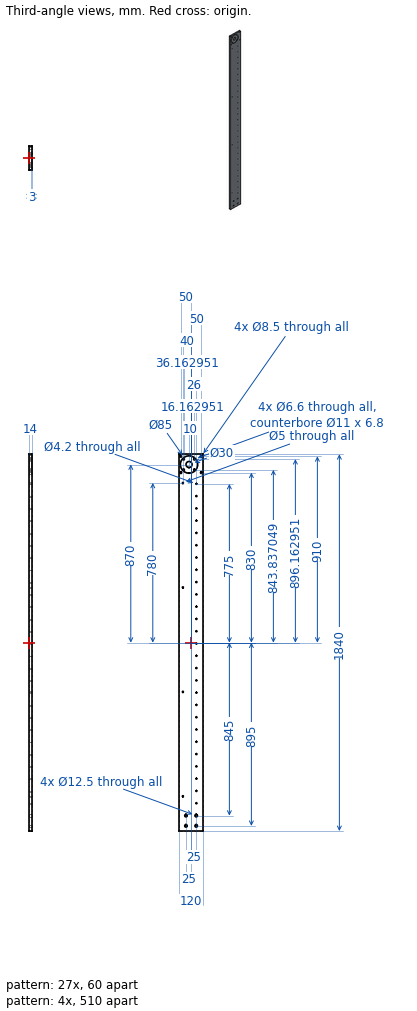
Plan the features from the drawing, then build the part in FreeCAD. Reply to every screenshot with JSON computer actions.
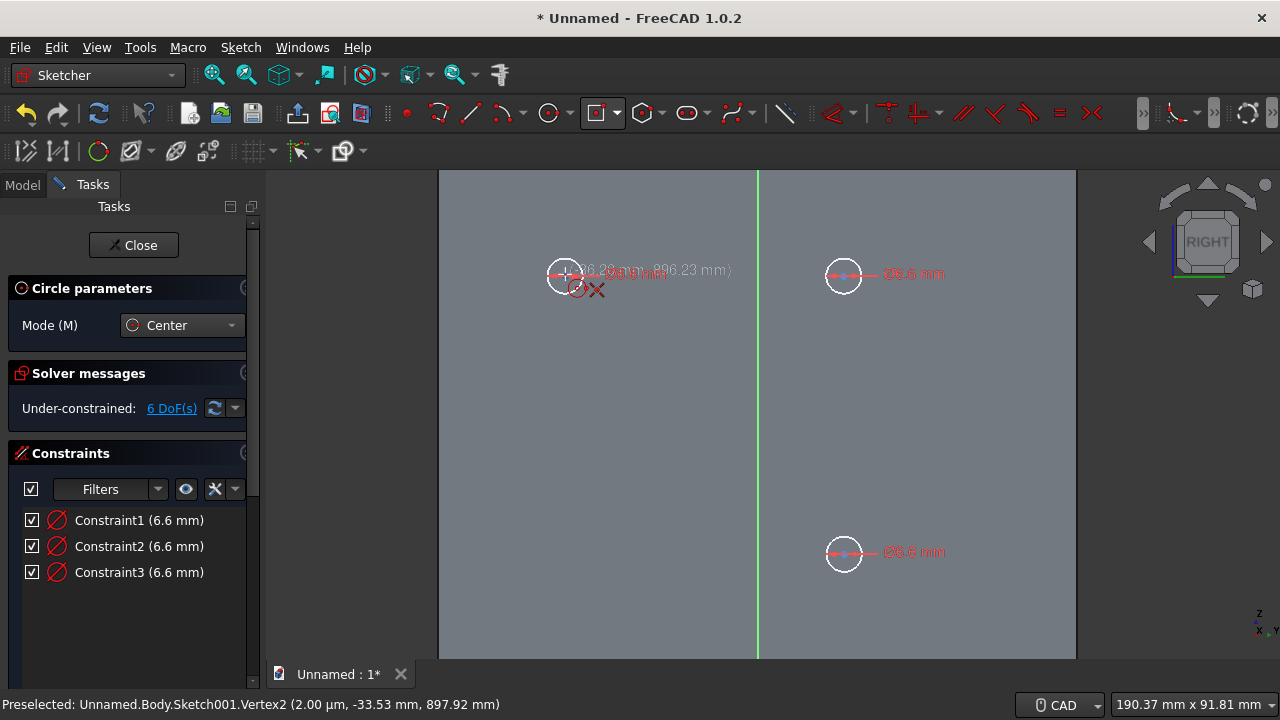
{"action": "scroll", "coordinate": [565, 554], "scroll_direction": "up", "scroll_amount": 2}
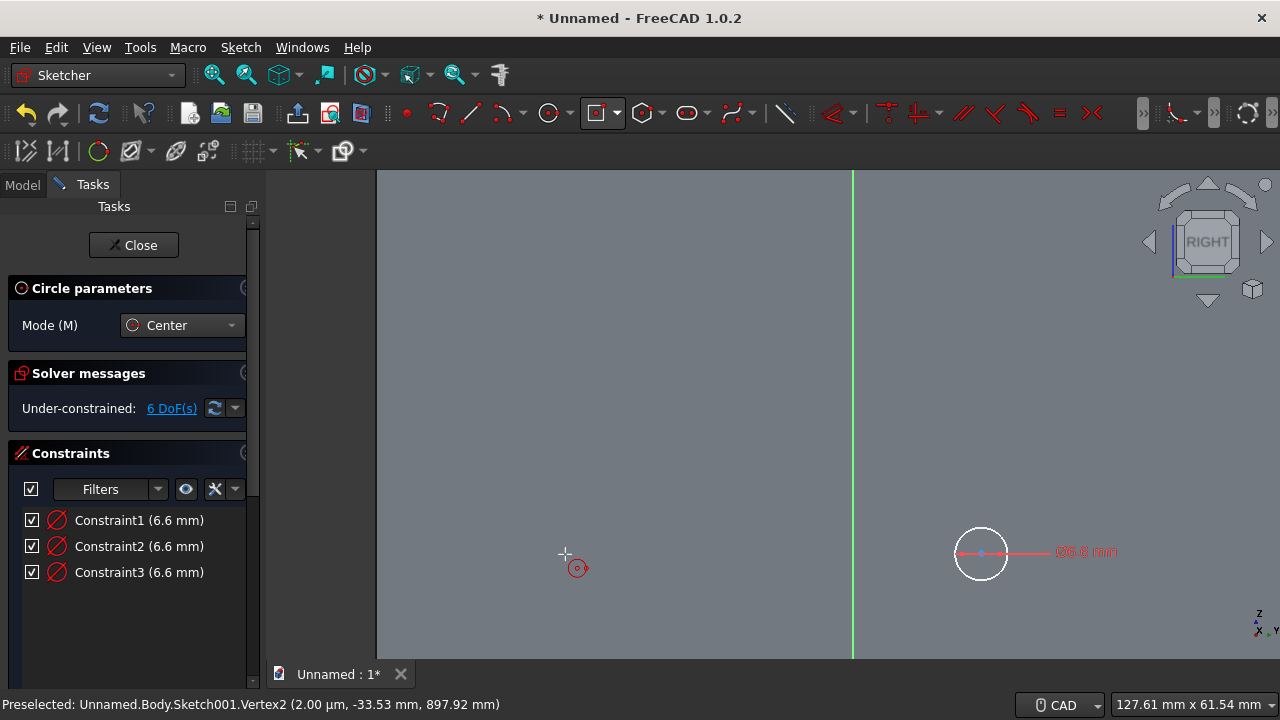
{"action": "left_click", "coordinate": [565, 553]}
{"action": "mouse_move", "coordinate": [584, 535]}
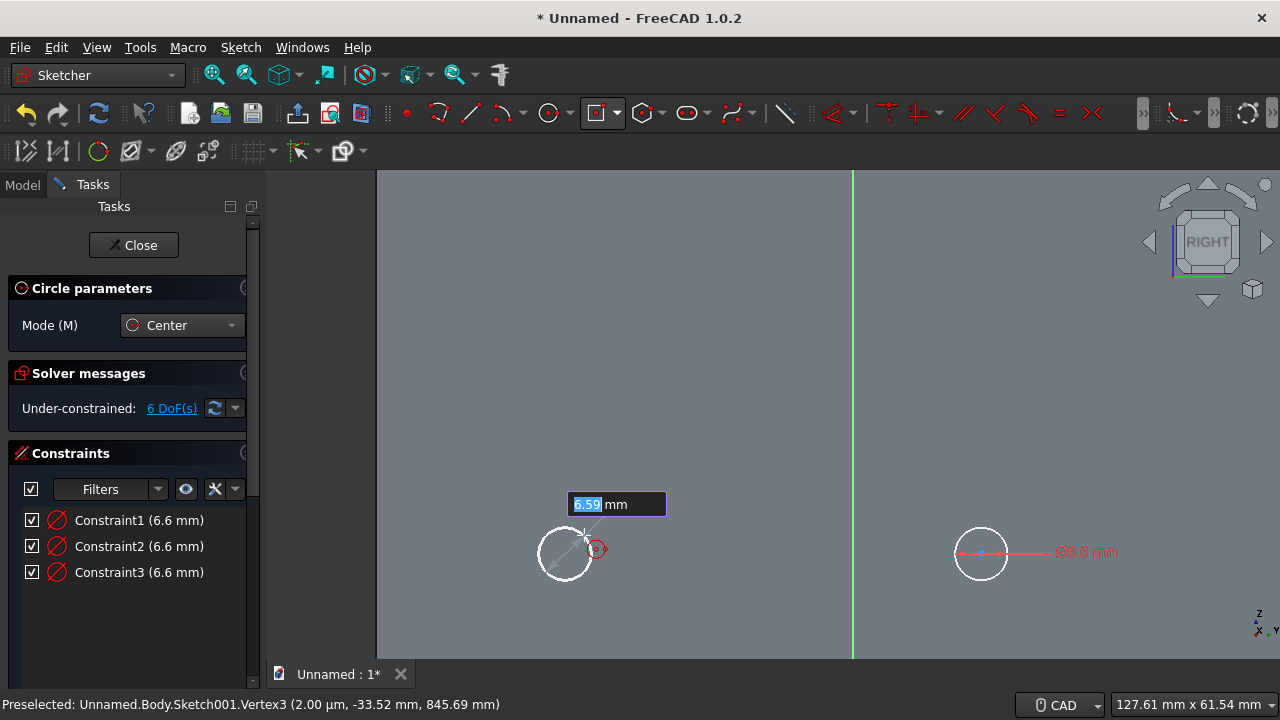
{"action": "type", "text": "6.6"}
{"action": "key", "text": "Return"}
{"action": "key", "text": "Escape"}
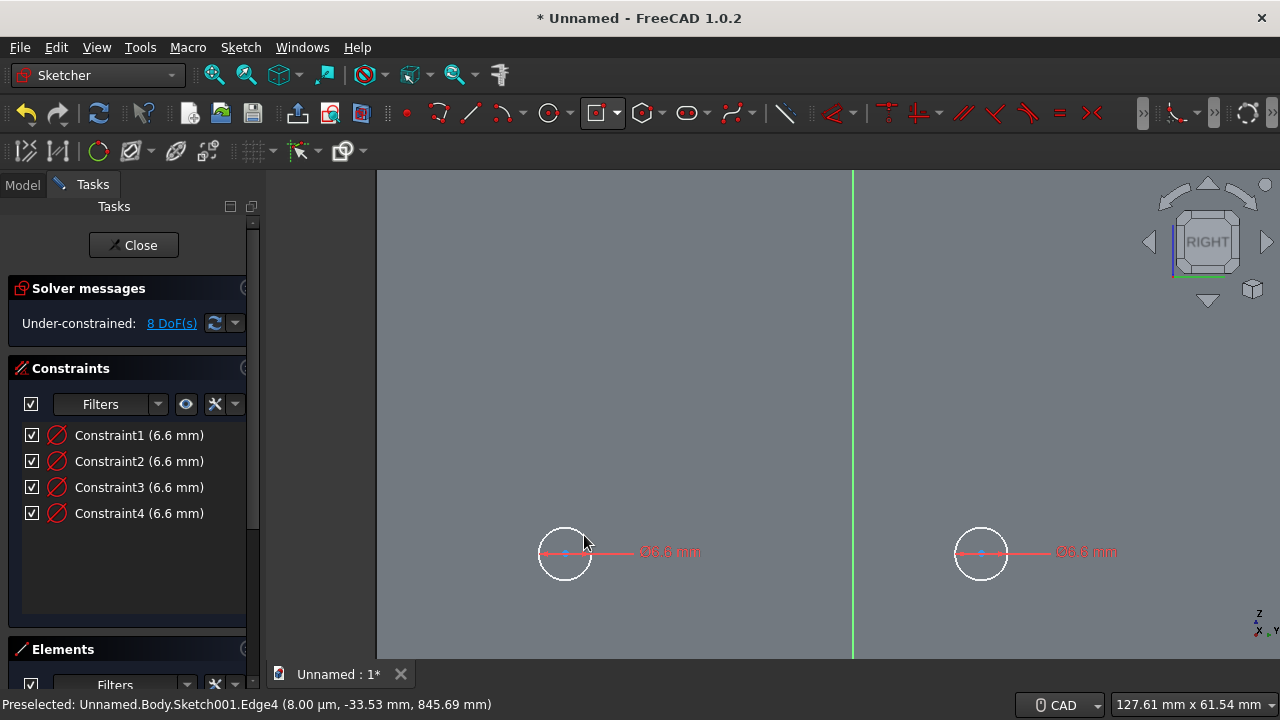
{"action": "scroll", "coordinate": [565, 555], "scroll_direction": "down", "scroll_amount": 2}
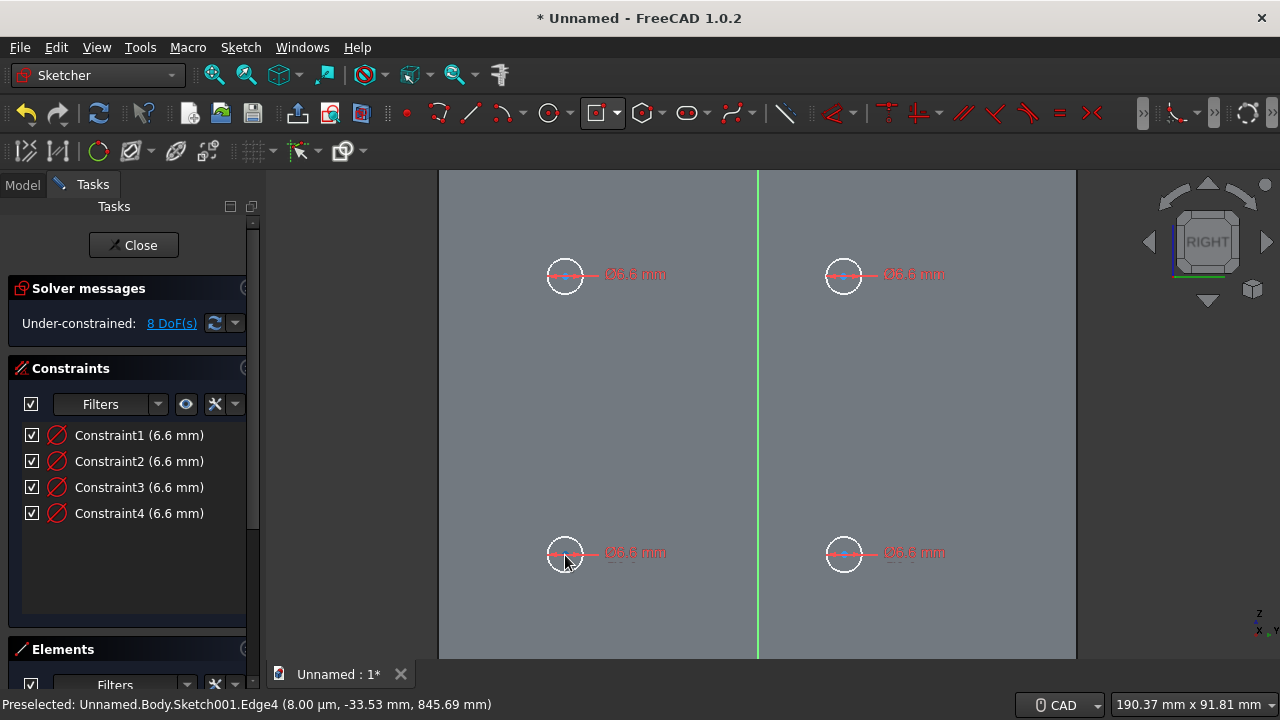
{"action": "left_click", "coordinate": [844, 276]}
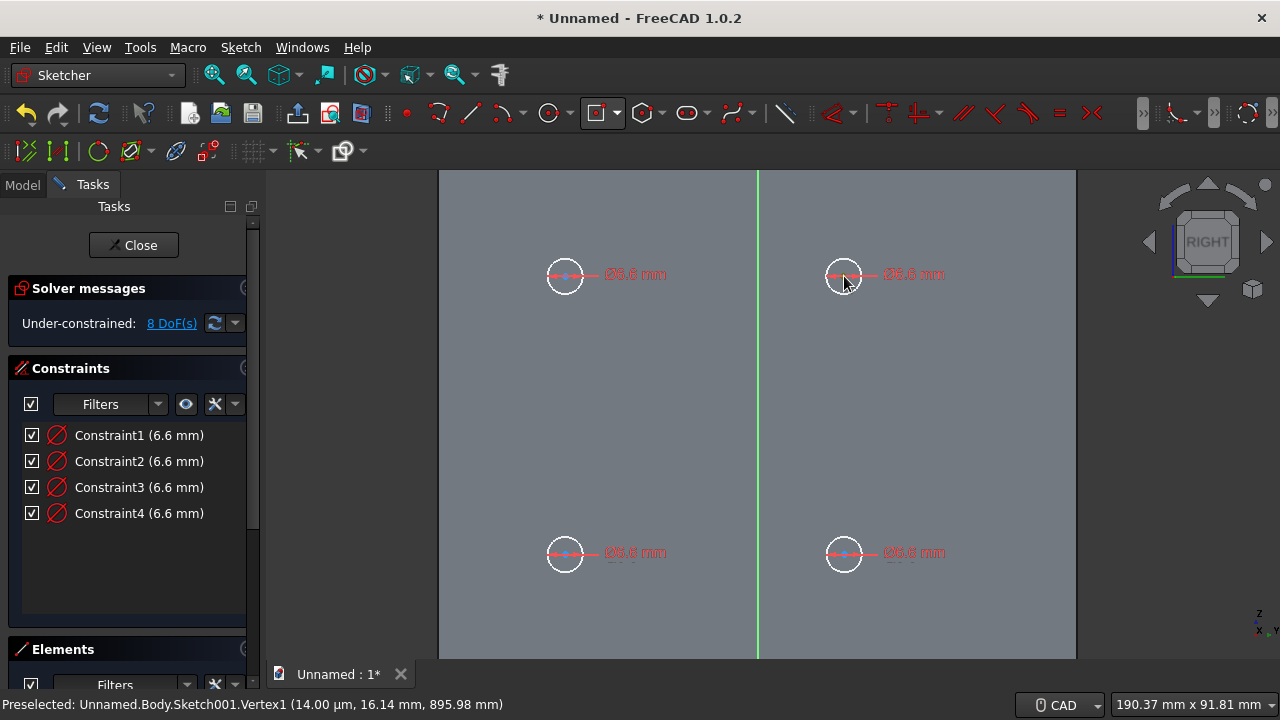
{"action": "left_click", "coordinate": [844, 555]}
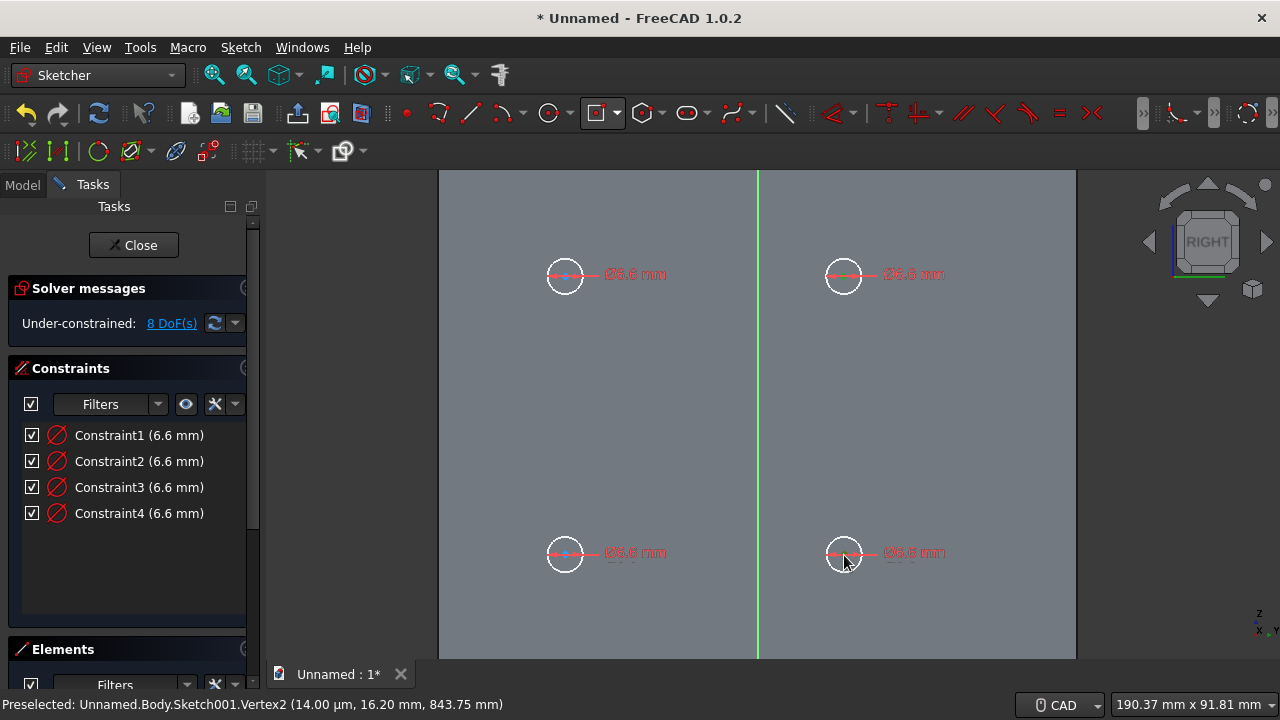
{"action": "key", "text": "v"}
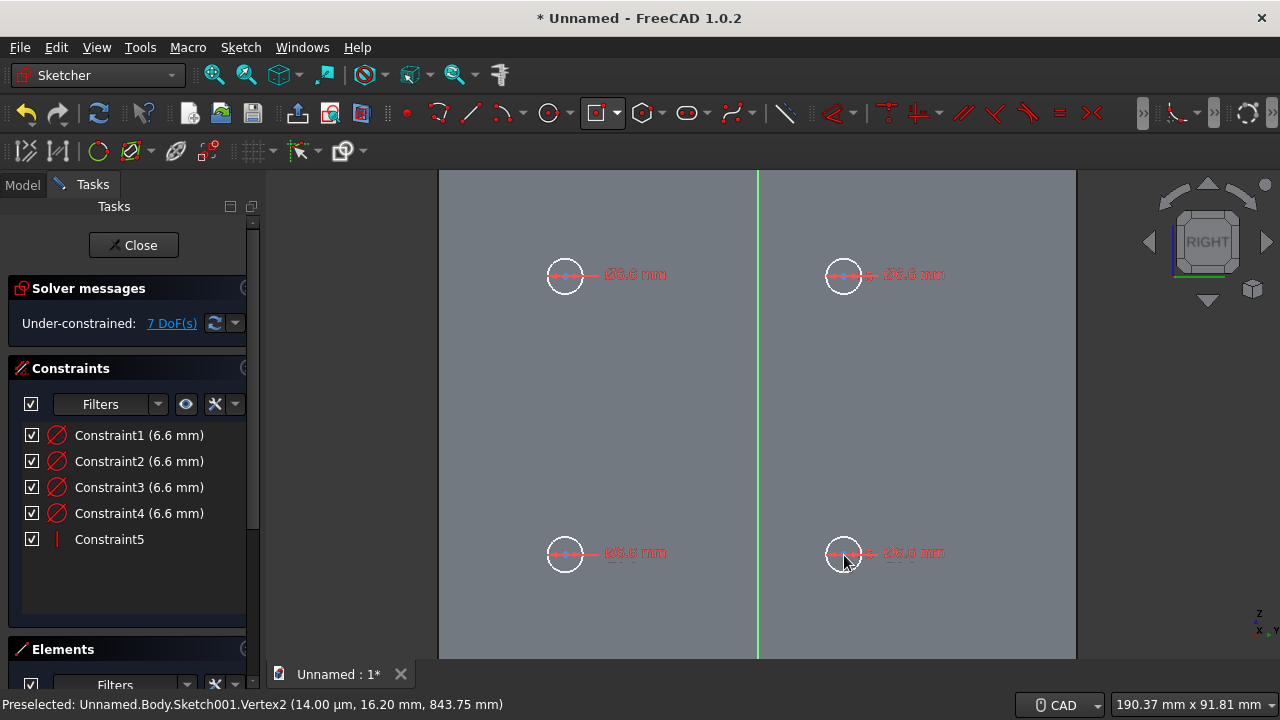
{"action": "left_click", "coordinate": [844, 276]}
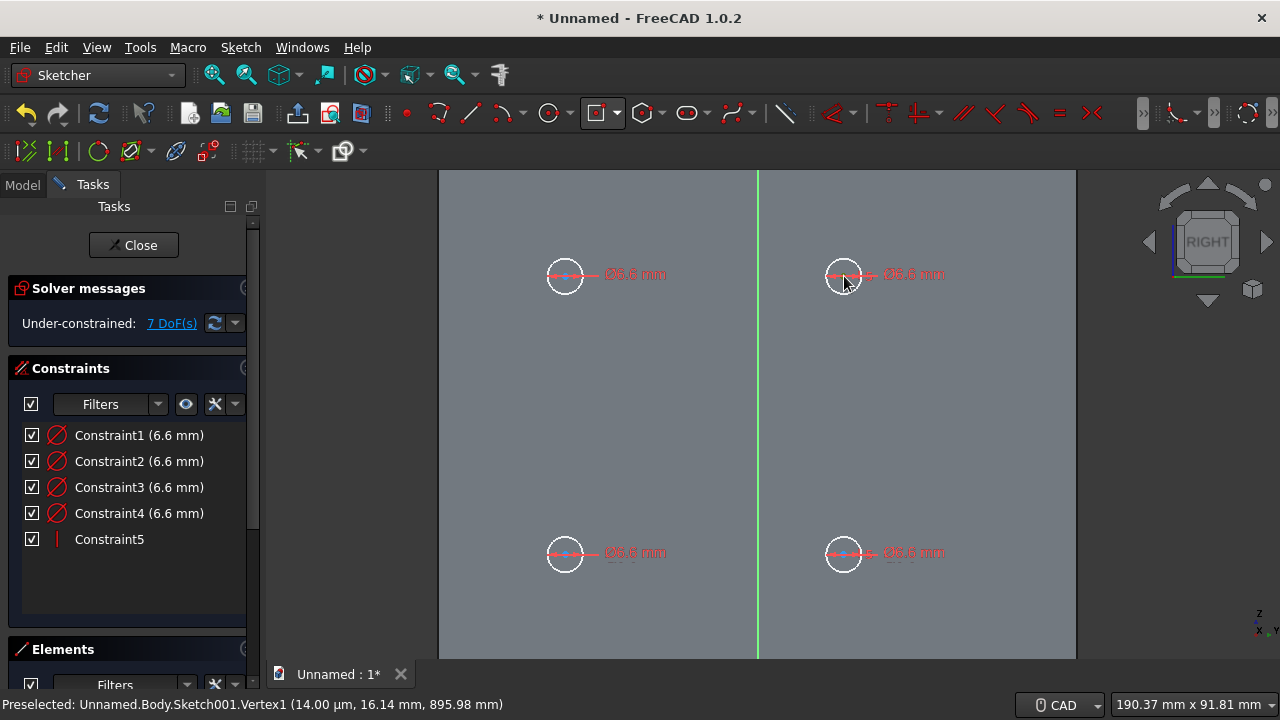
{"action": "left_click", "coordinate": [565, 276]}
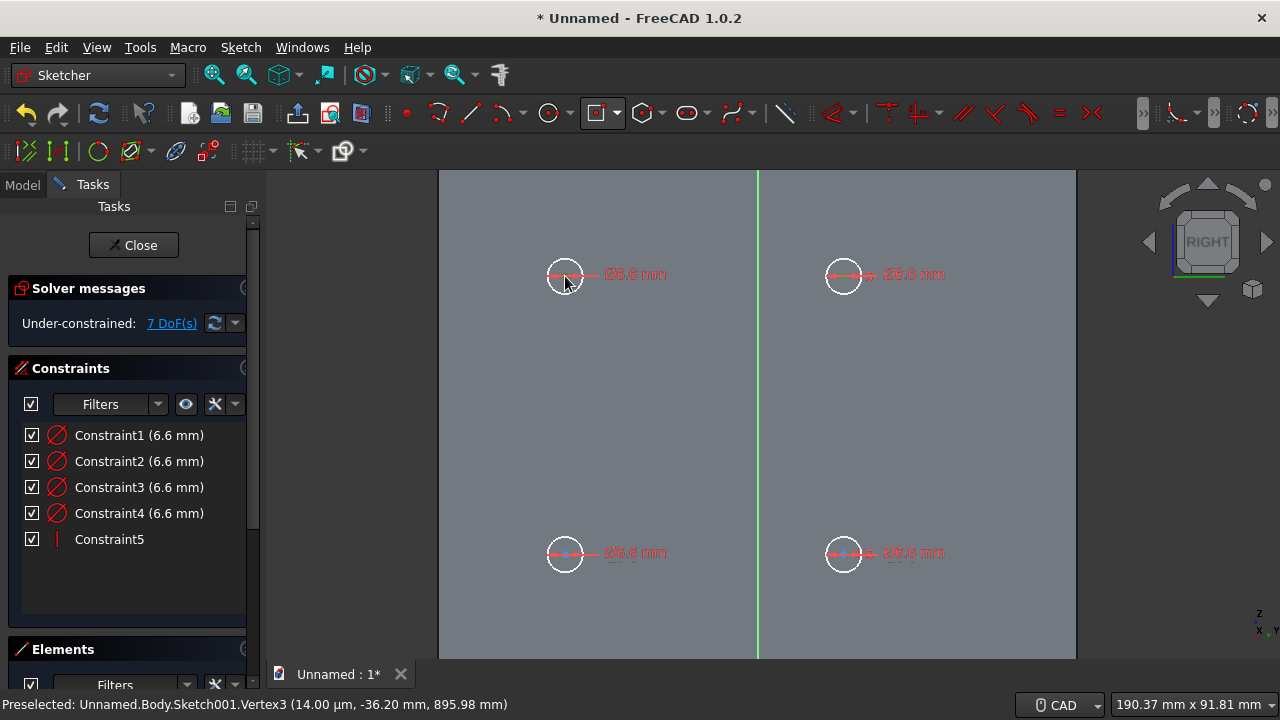
{"action": "key", "text": "h"}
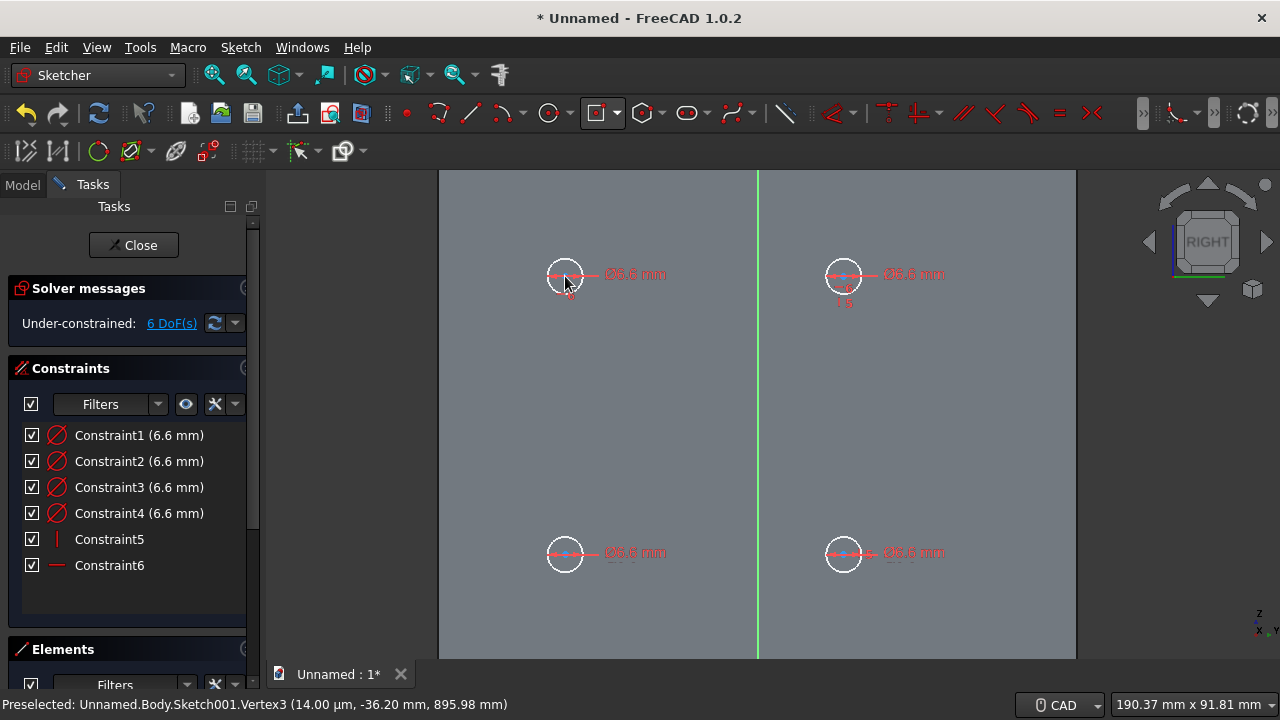
{"action": "left_click", "coordinate": [565, 276]}